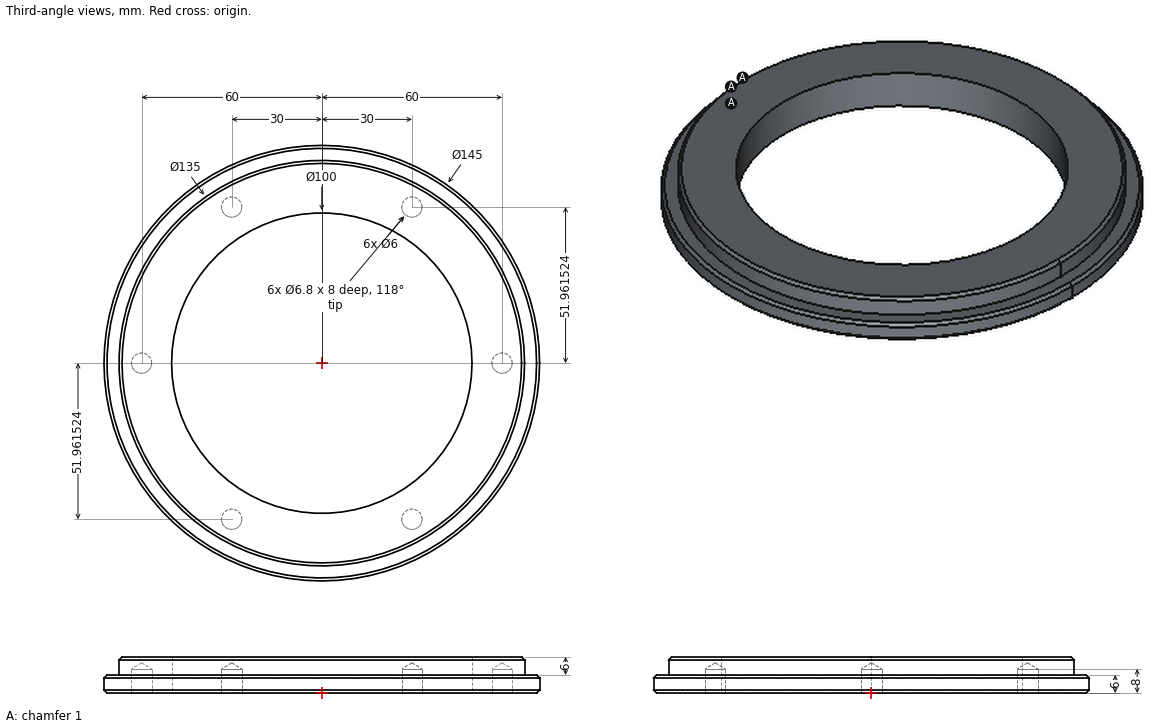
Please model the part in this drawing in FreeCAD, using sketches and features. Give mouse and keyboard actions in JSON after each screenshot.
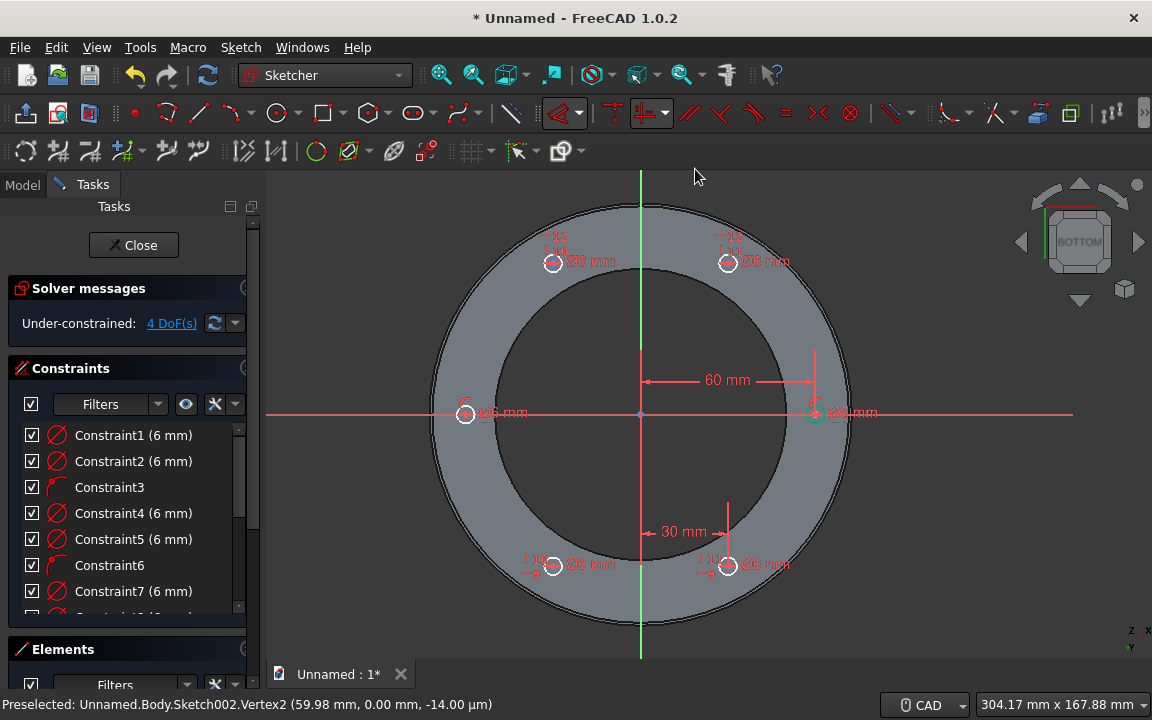
{"action": "left_click", "coordinate": [553, 566]}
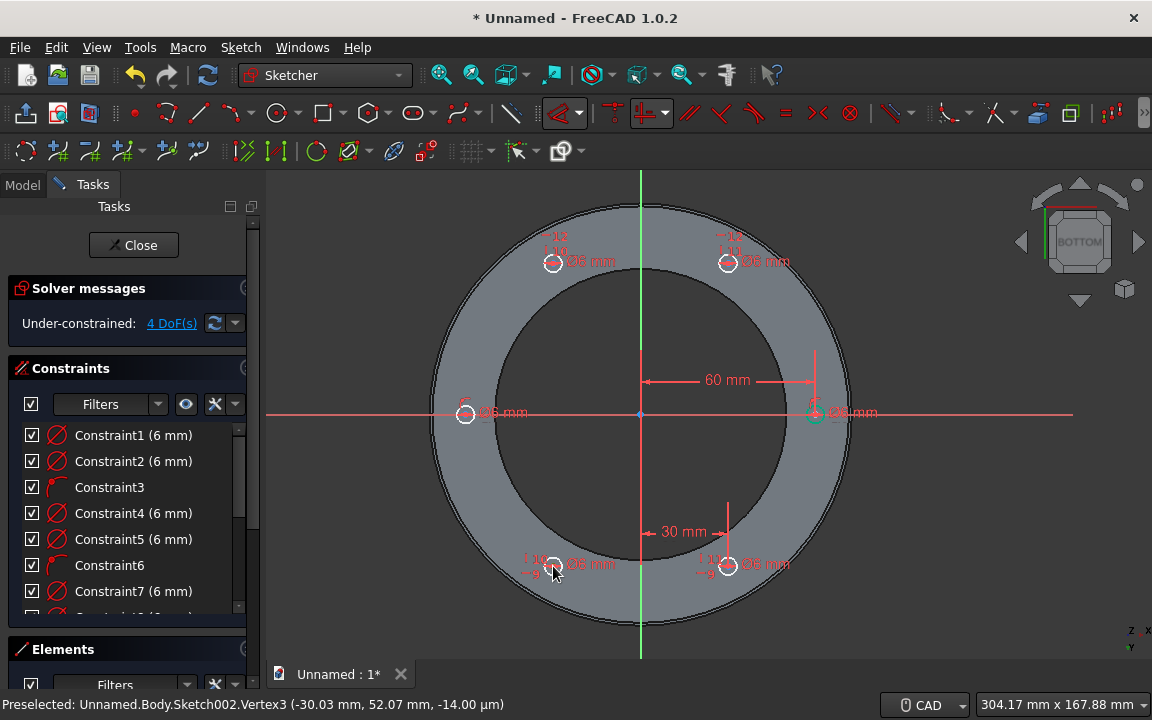
{"action": "left_click", "coordinate": [582, 114]}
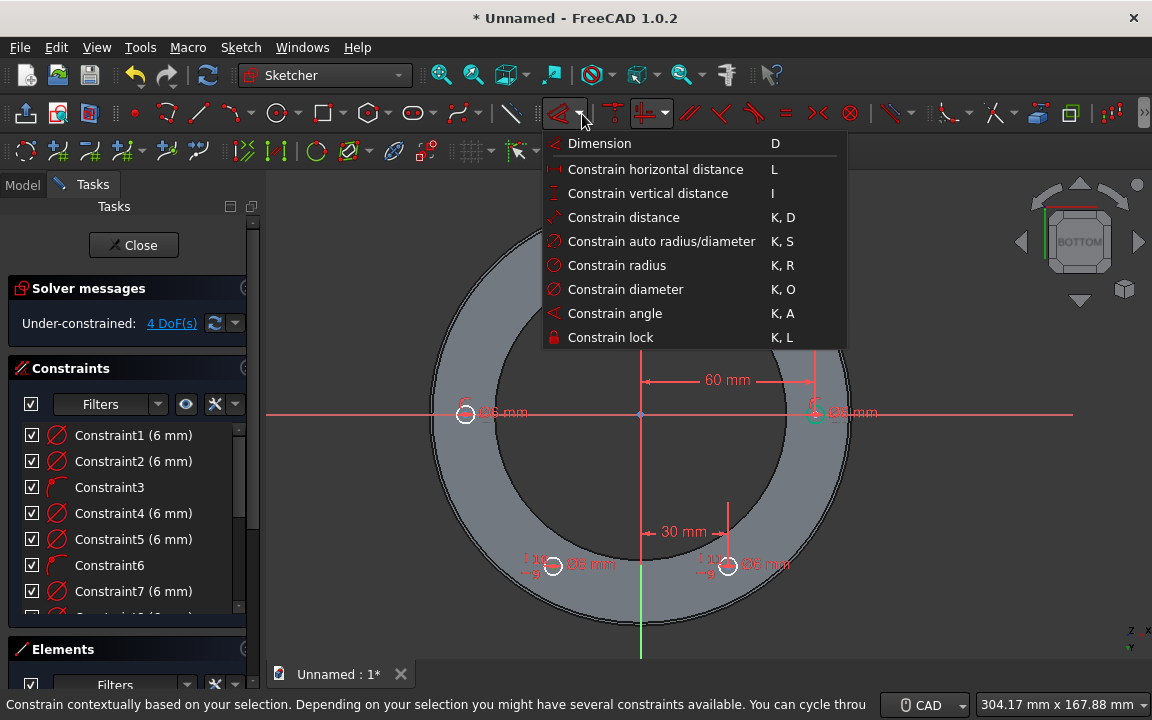
{"action": "left_click", "coordinate": [695, 169]}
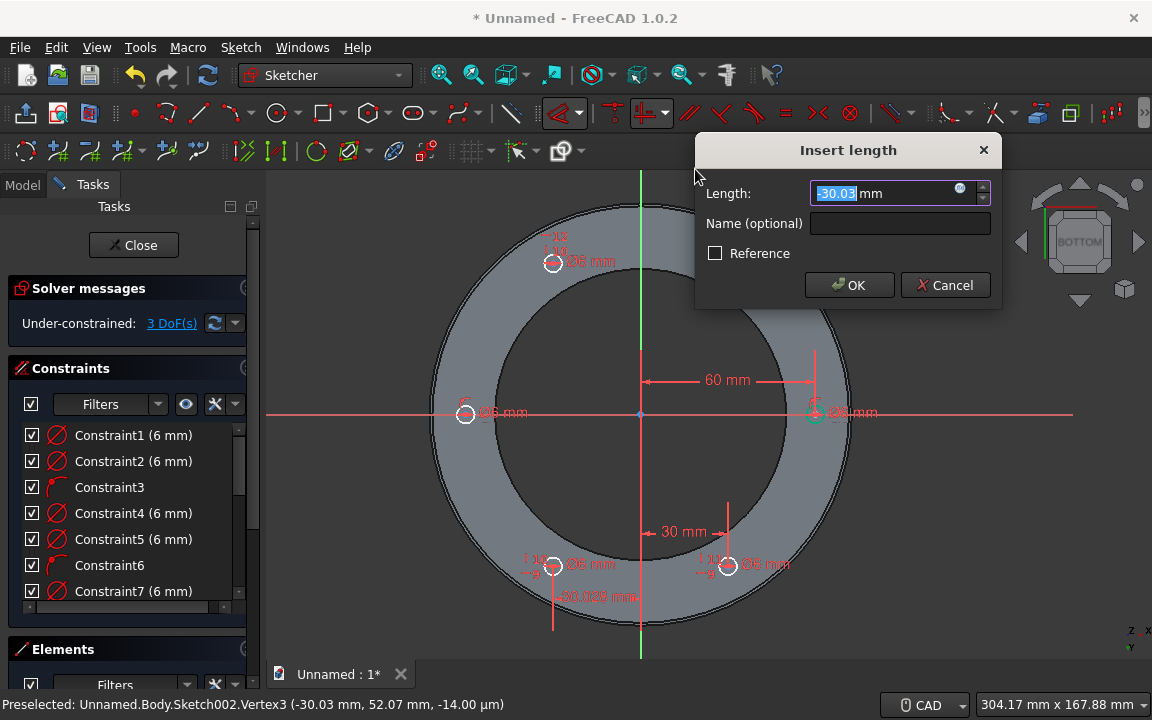
{"action": "type", "text": "-30"}
{"action": "key", "text": "Return"}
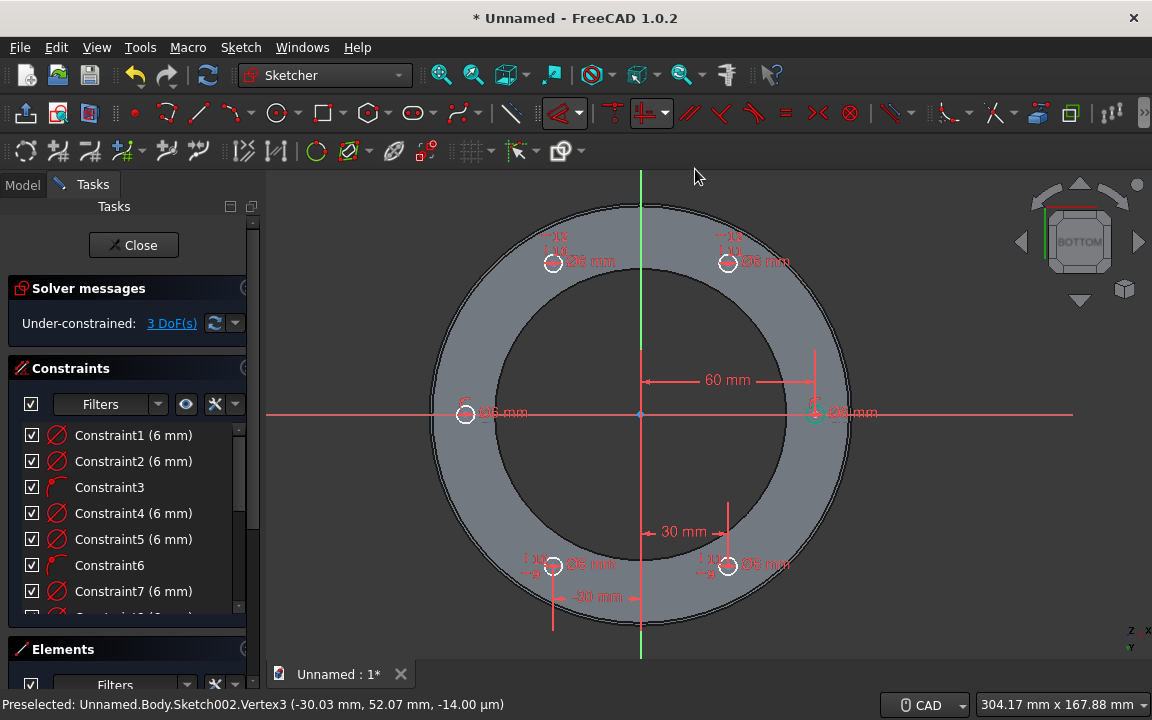
{"action": "left_click", "coordinate": [466, 415]}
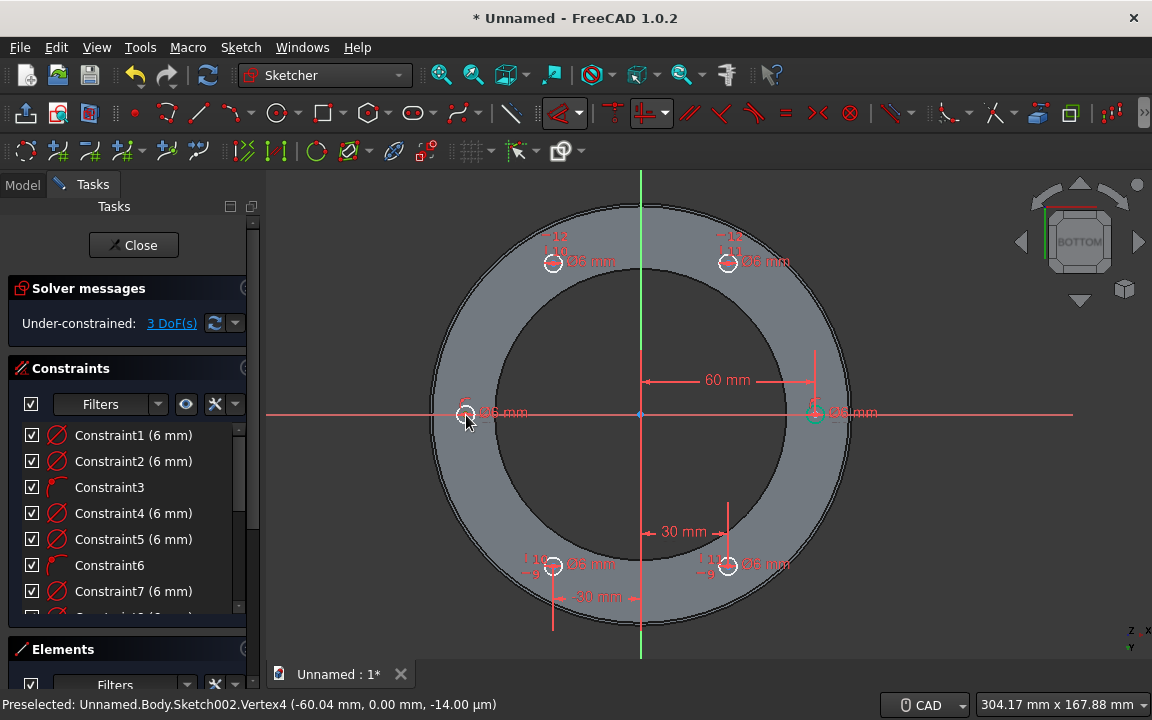
{"action": "left_click", "coordinate": [582, 114]}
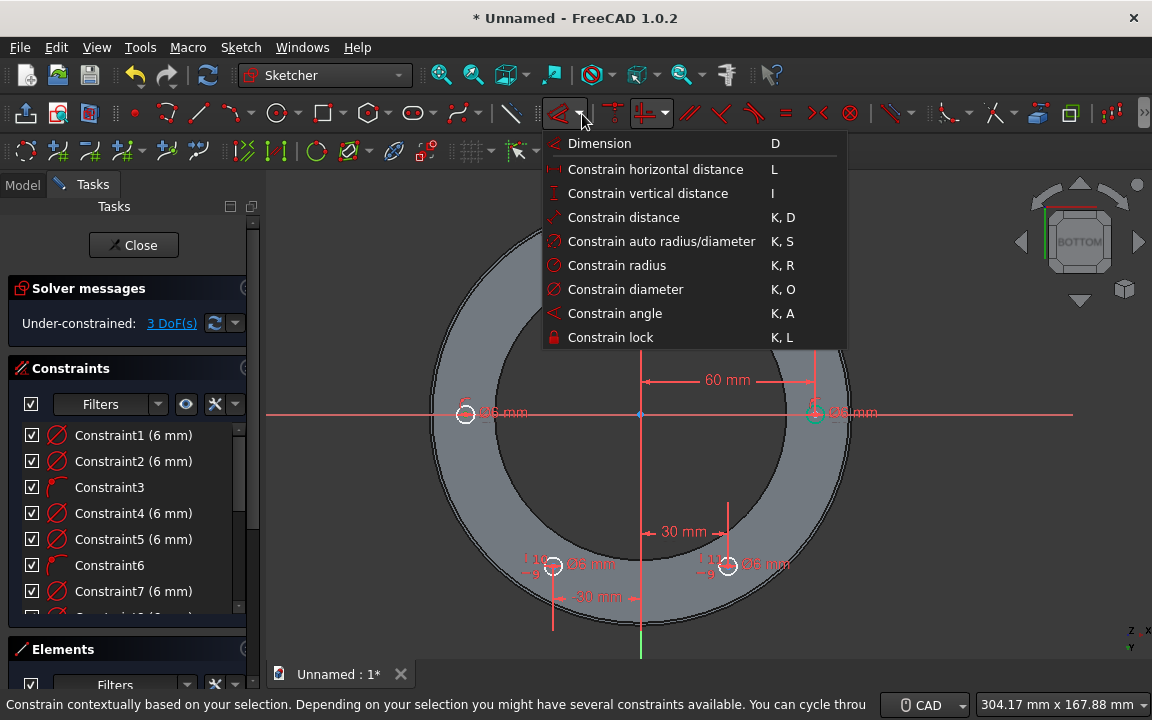
{"action": "left_click", "coordinate": [695, 169]}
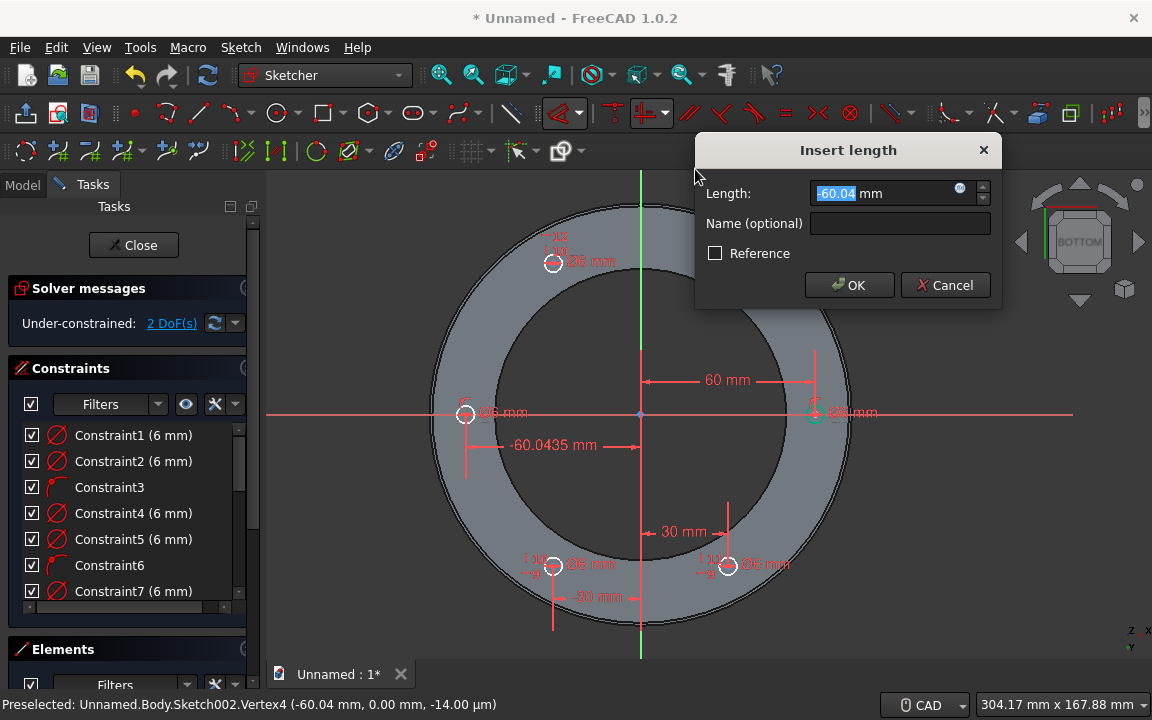
{"action": "type", "text": "-60"}
{"action": "key", "text": "Return"}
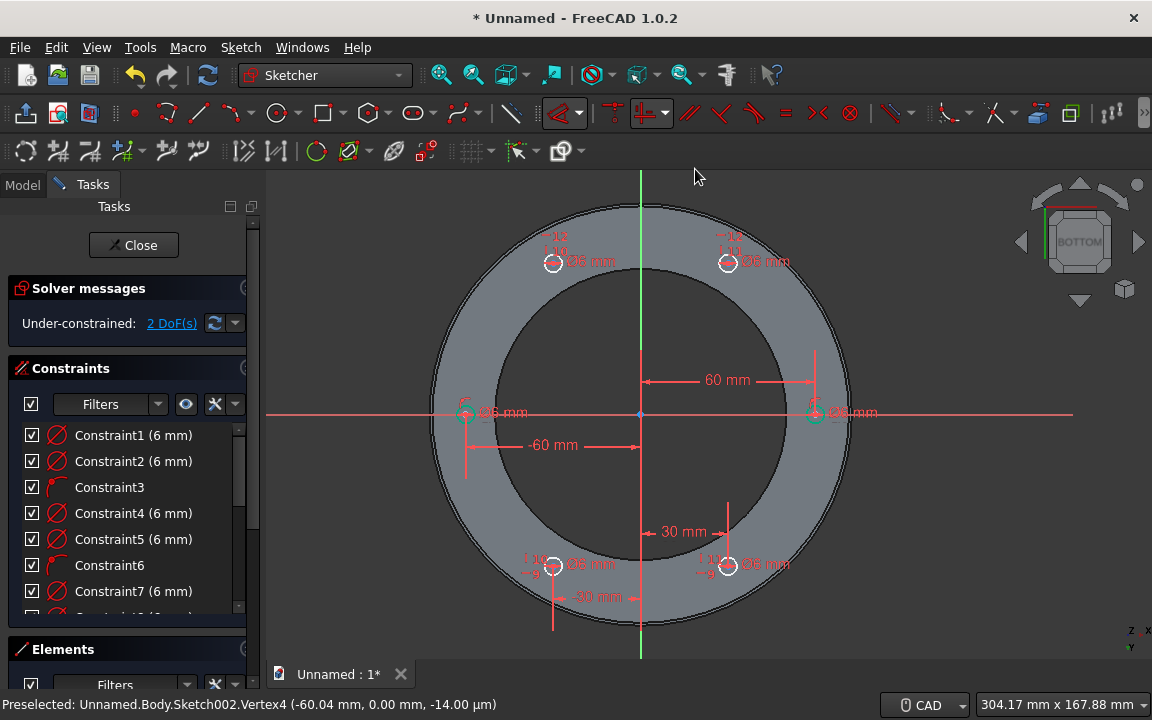
{"action": "left_click", "coordinate": [728, 566]}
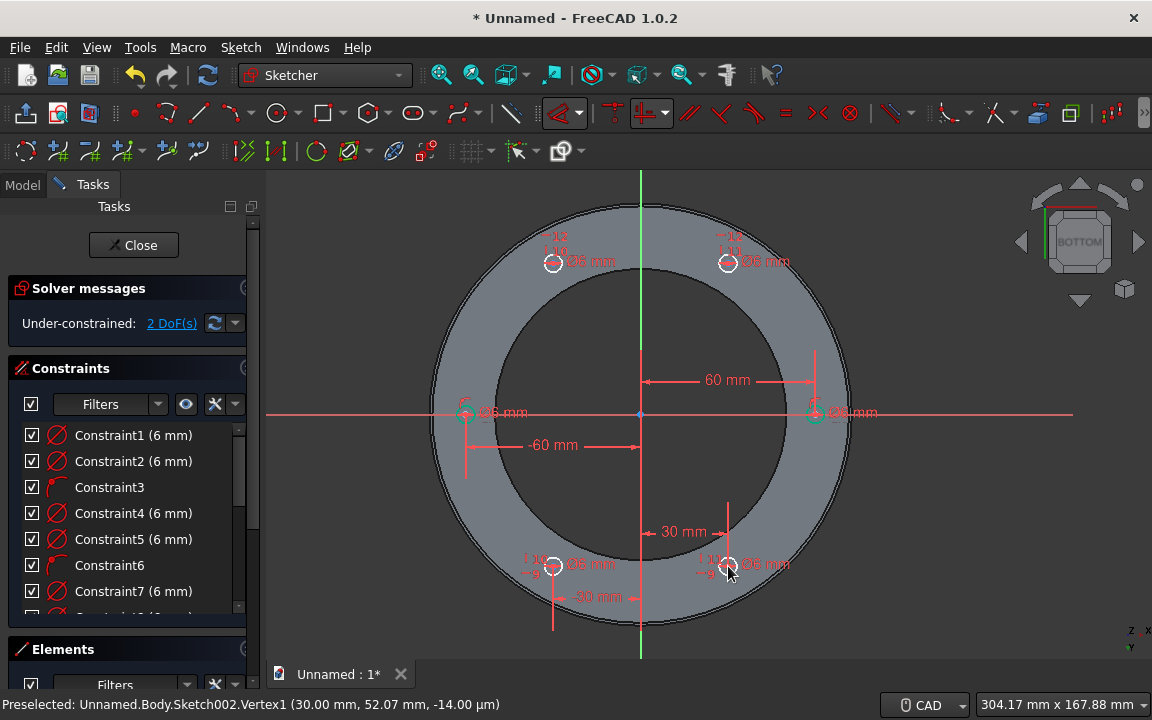
{"action": "left_click", "coordinate": [582, 114]}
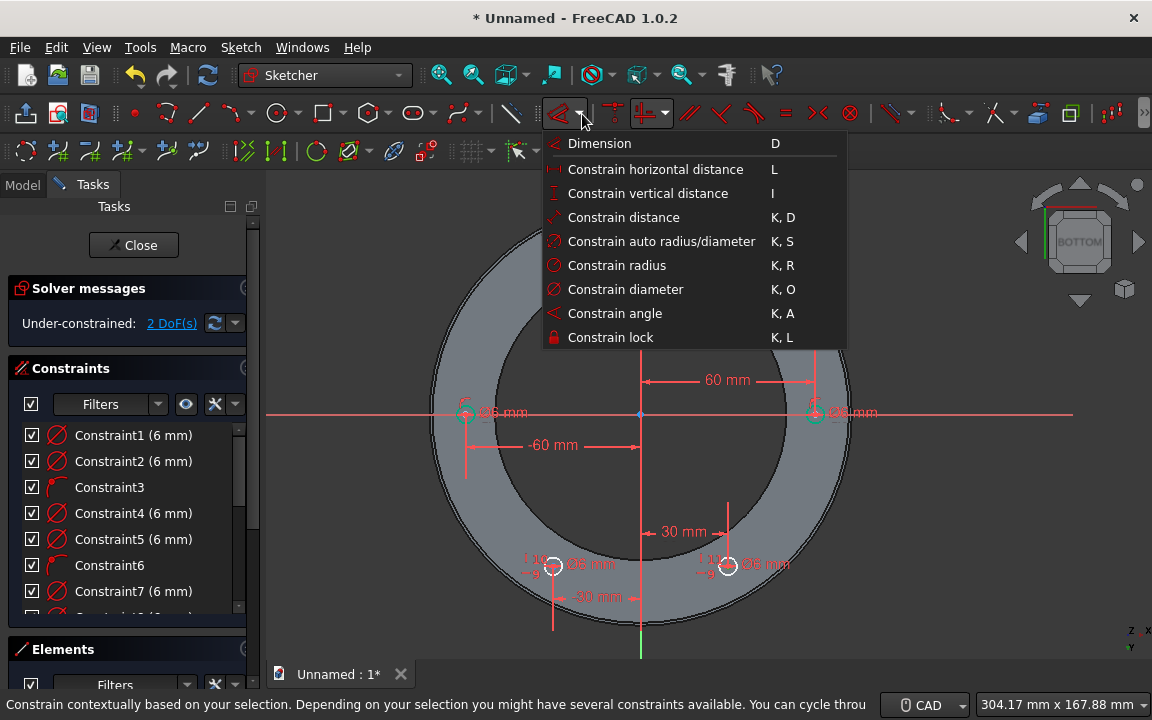
{"action": "left_click", "coordinate": [695, 193]}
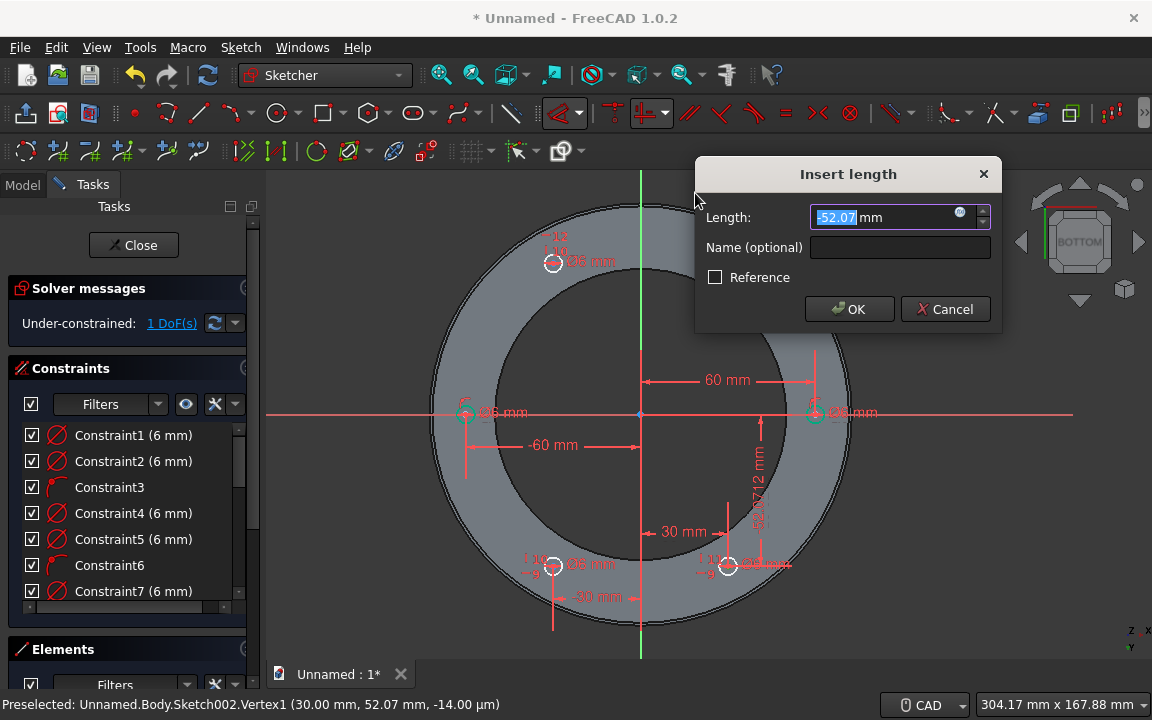
{"action": "type", "text": "-51.961524"}
{"action": "key", "text": "Return"}